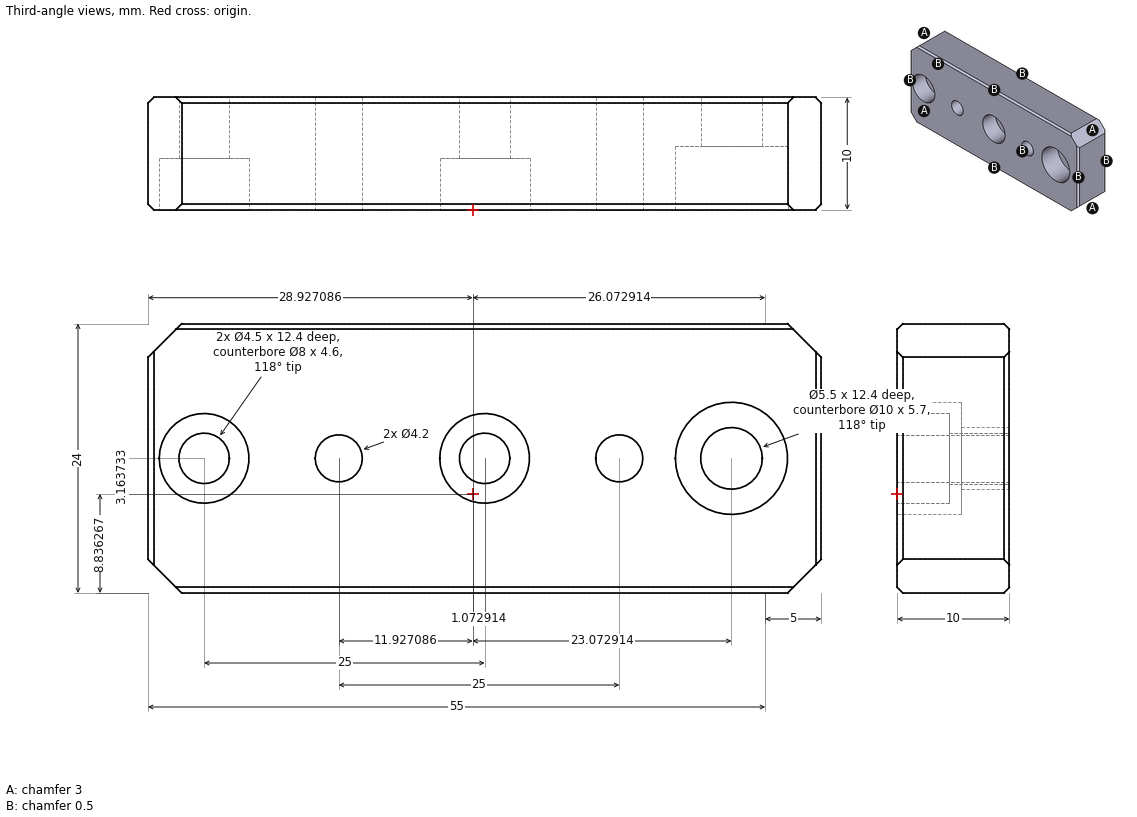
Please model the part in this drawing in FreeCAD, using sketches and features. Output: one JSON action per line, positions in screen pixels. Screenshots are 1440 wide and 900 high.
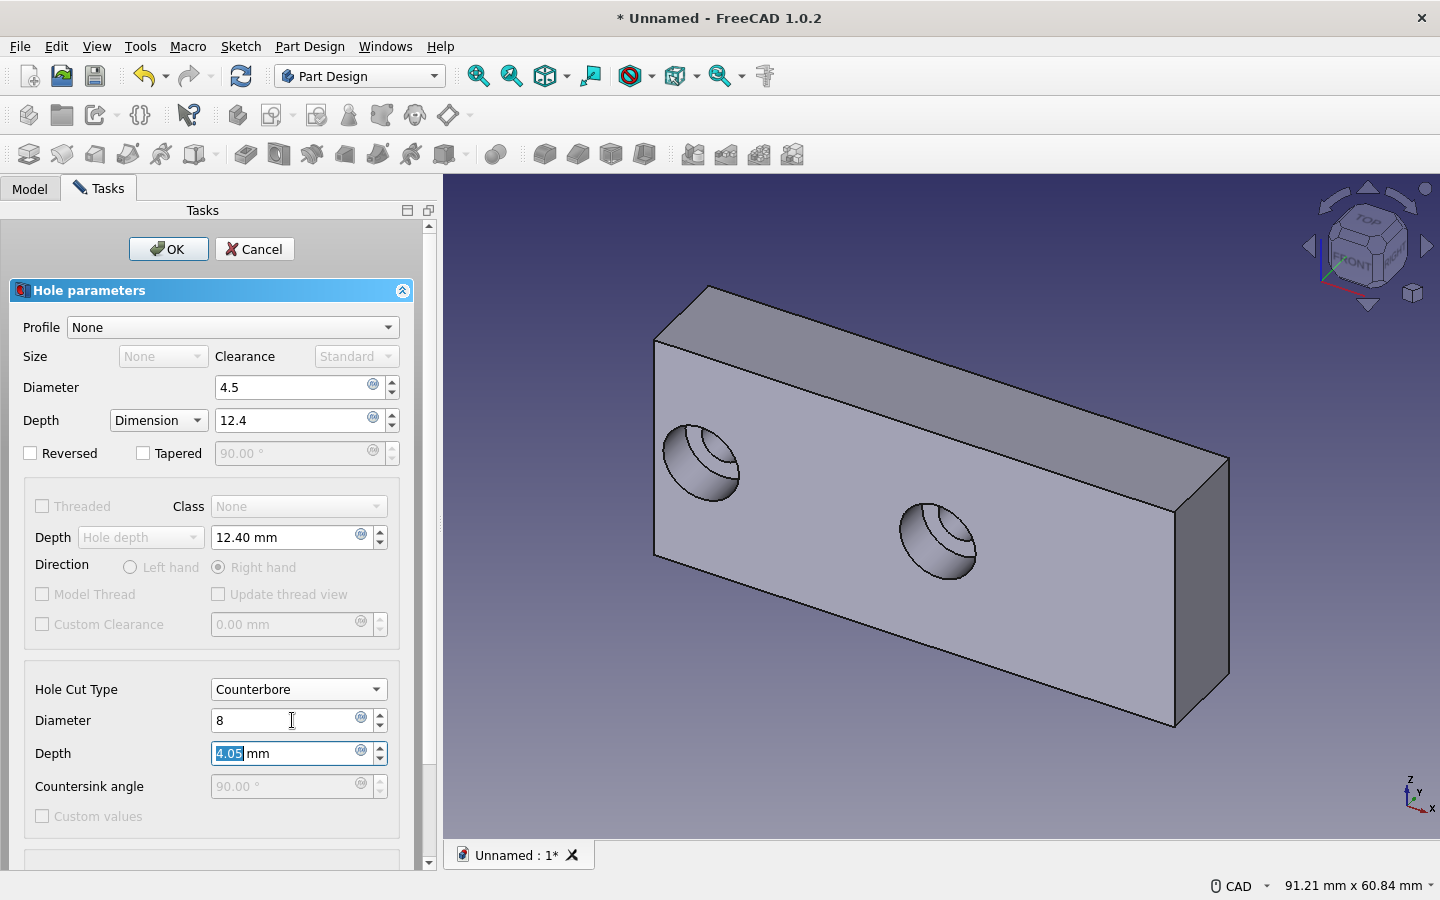
{"action": "type", "text": "4.6"}
{"action": "key", "text": "Tab"}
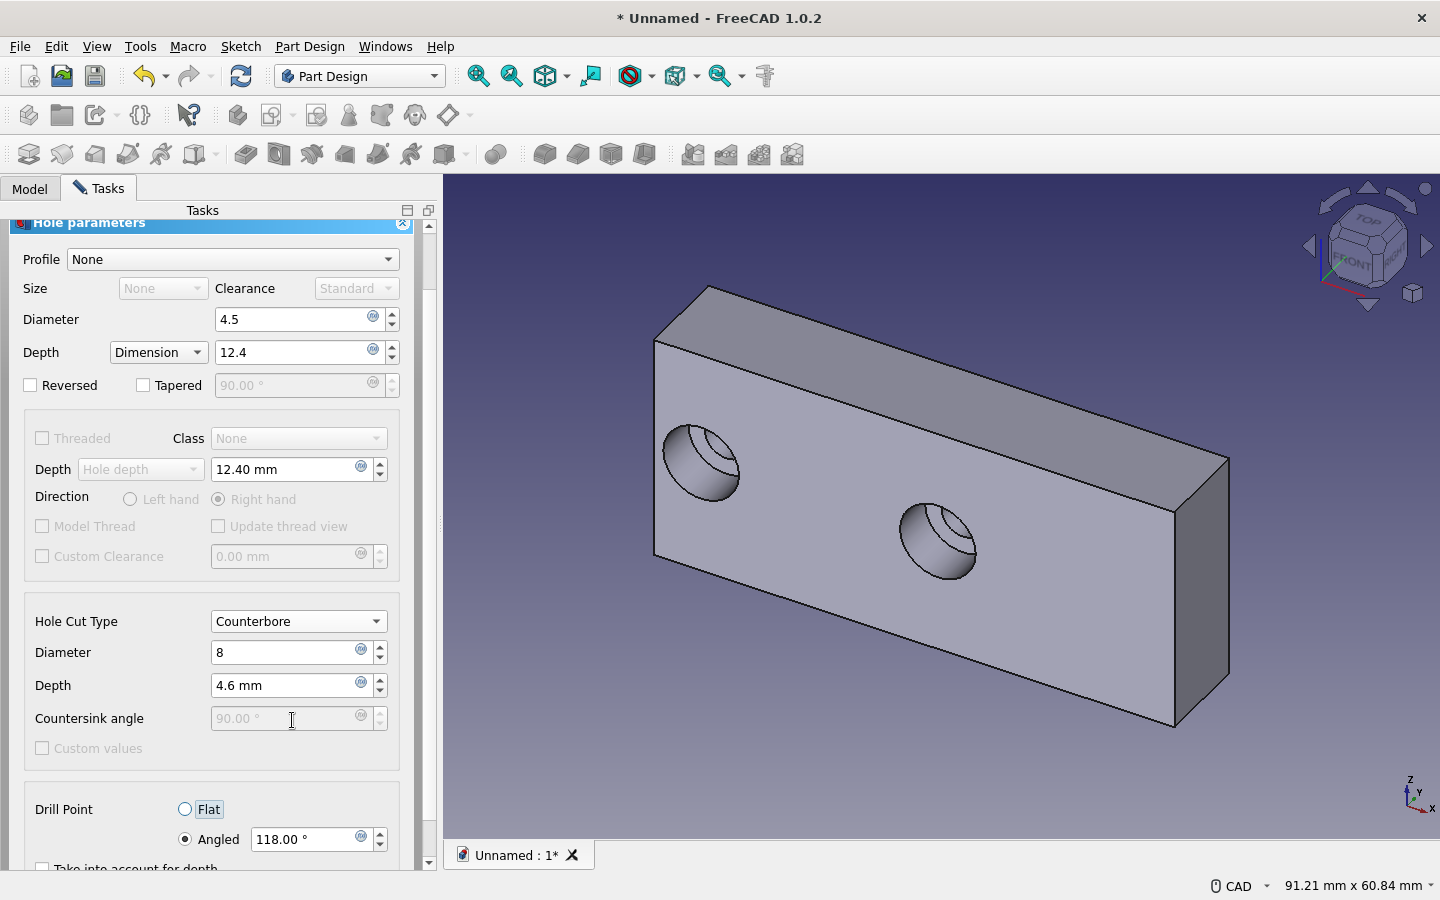
{"action": "scroll", "coordinate": [429, 545], "scroll_direction": "up", "scroll_amount": 2}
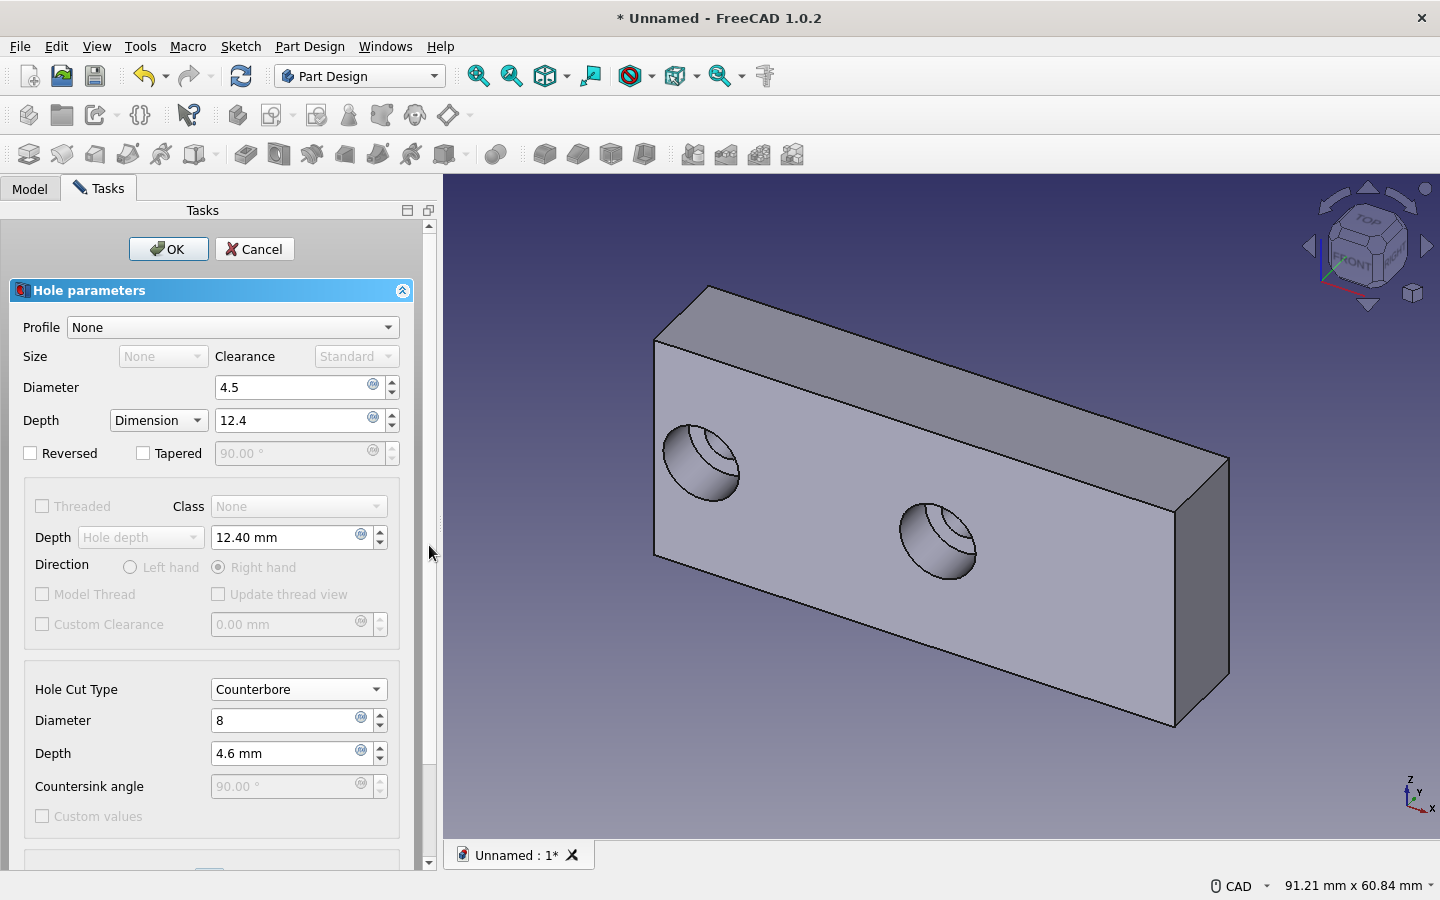
{"action": "left_click", "coordinate": [169, 249]}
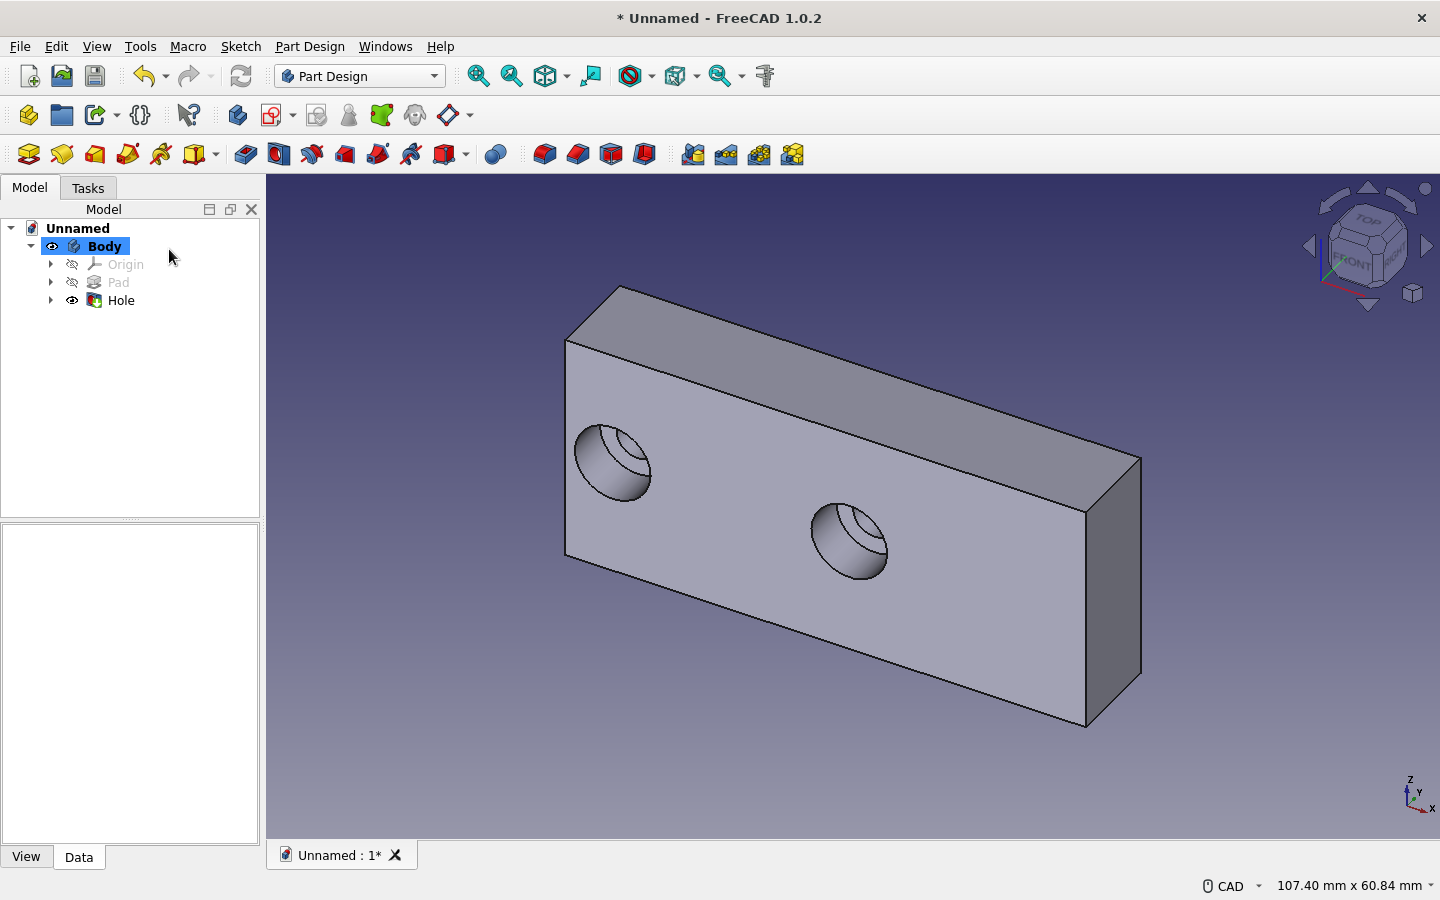
{"action": "left_click", "coordinate": [974, 582]}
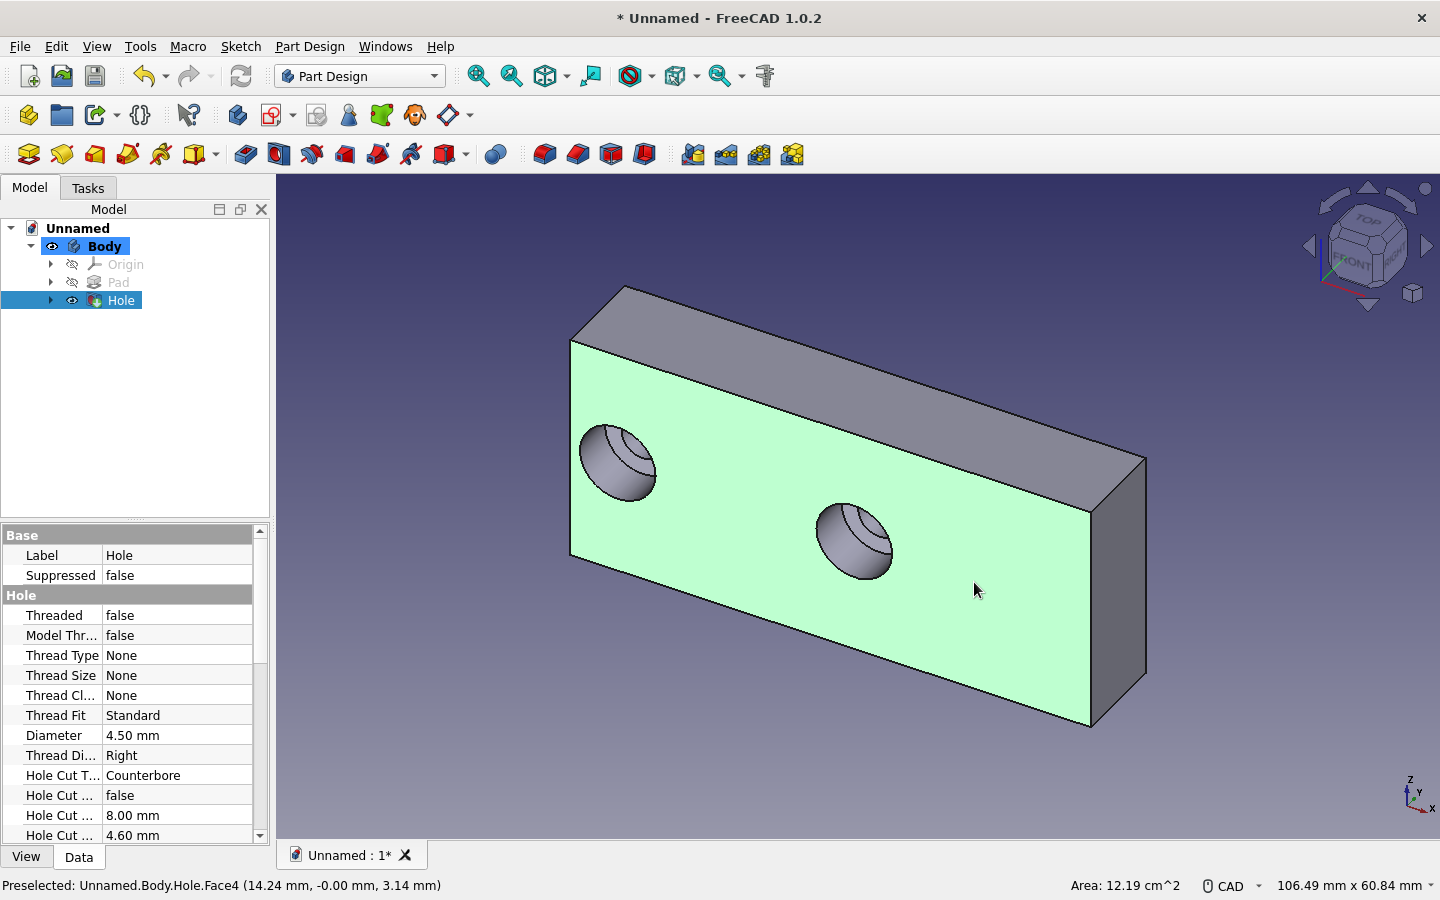
{"action": "left_click", "coordinate": [270, 116]}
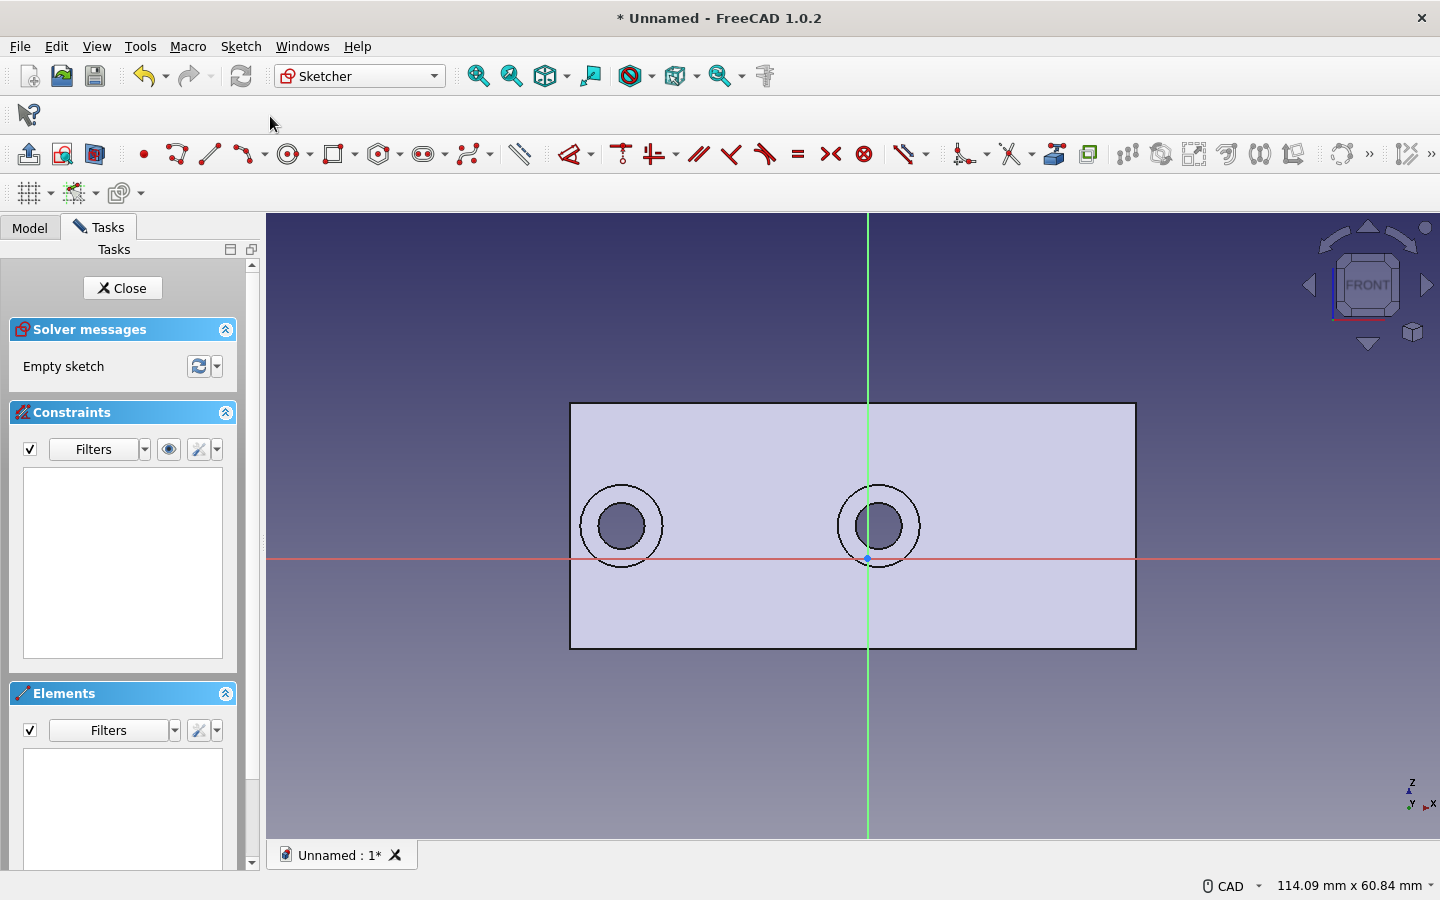
{"action": "scroll", "coordinate": [1275, 526], "scroll_direction": "up", "scroll_amount": 2}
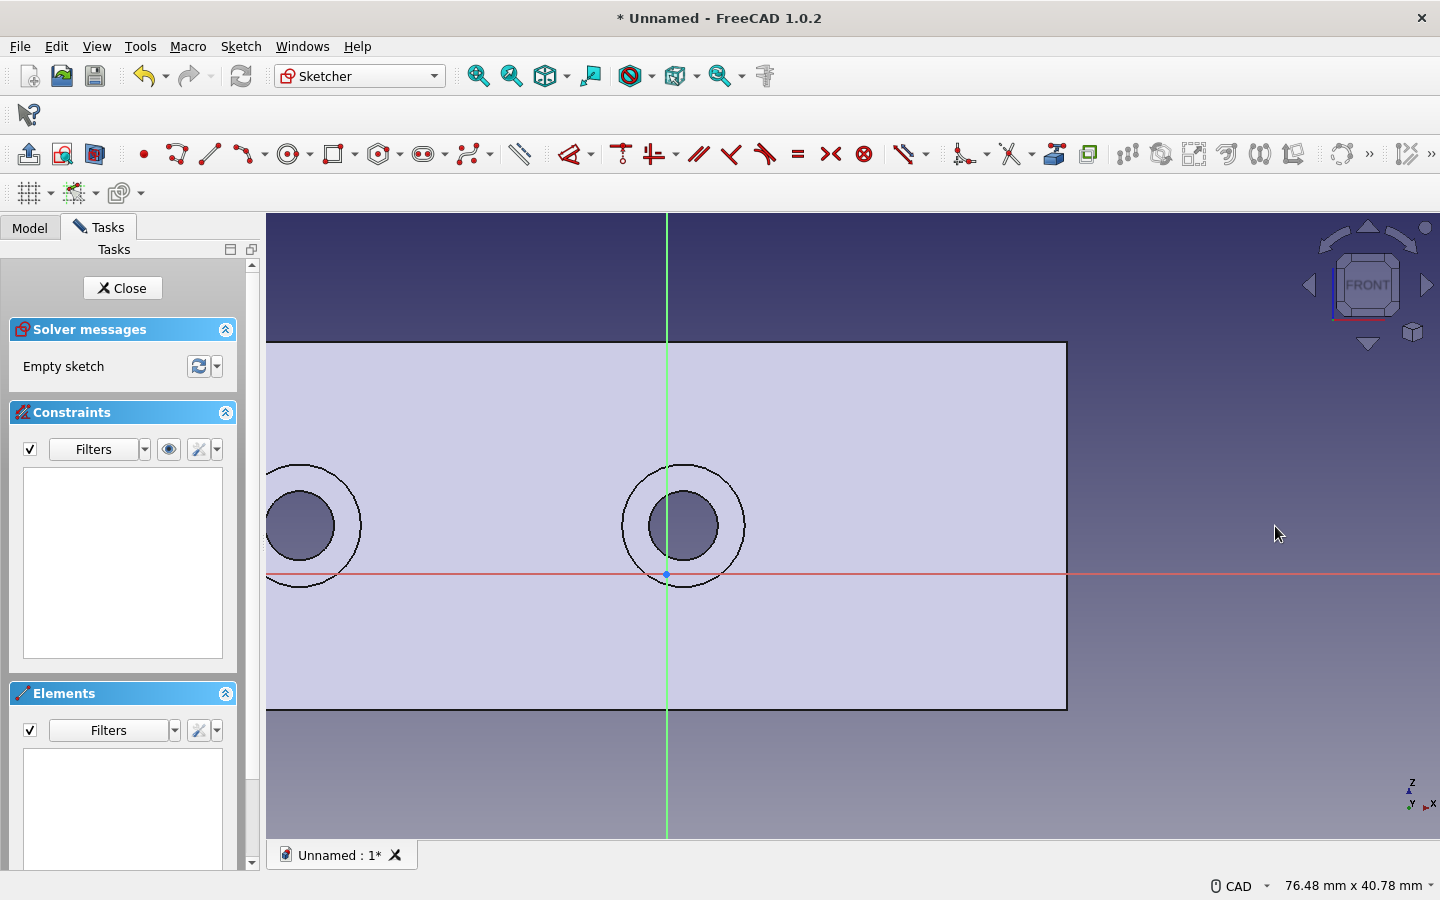
{"action": "key", "text": "g r"}